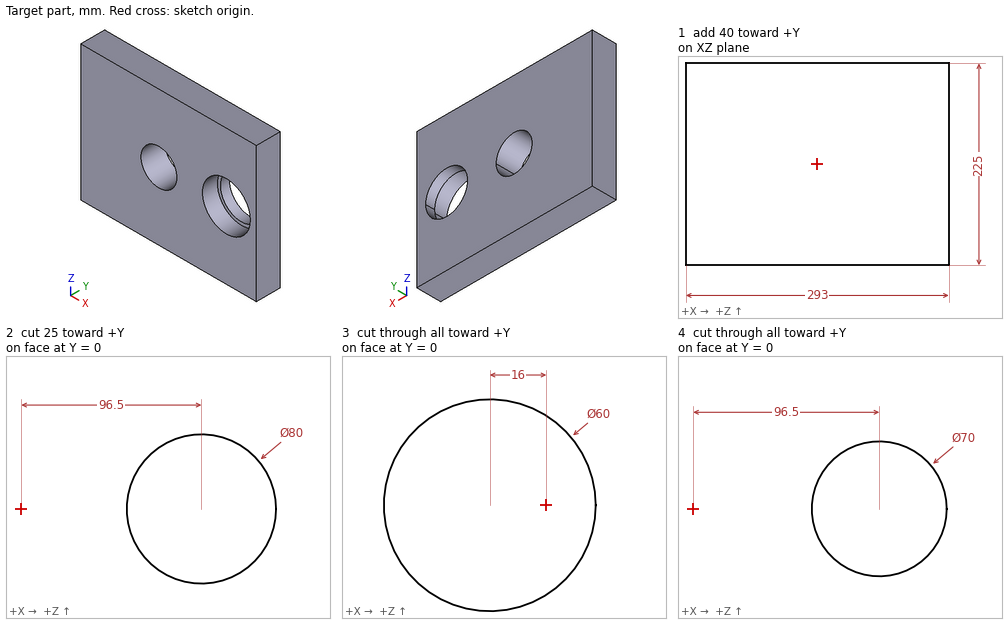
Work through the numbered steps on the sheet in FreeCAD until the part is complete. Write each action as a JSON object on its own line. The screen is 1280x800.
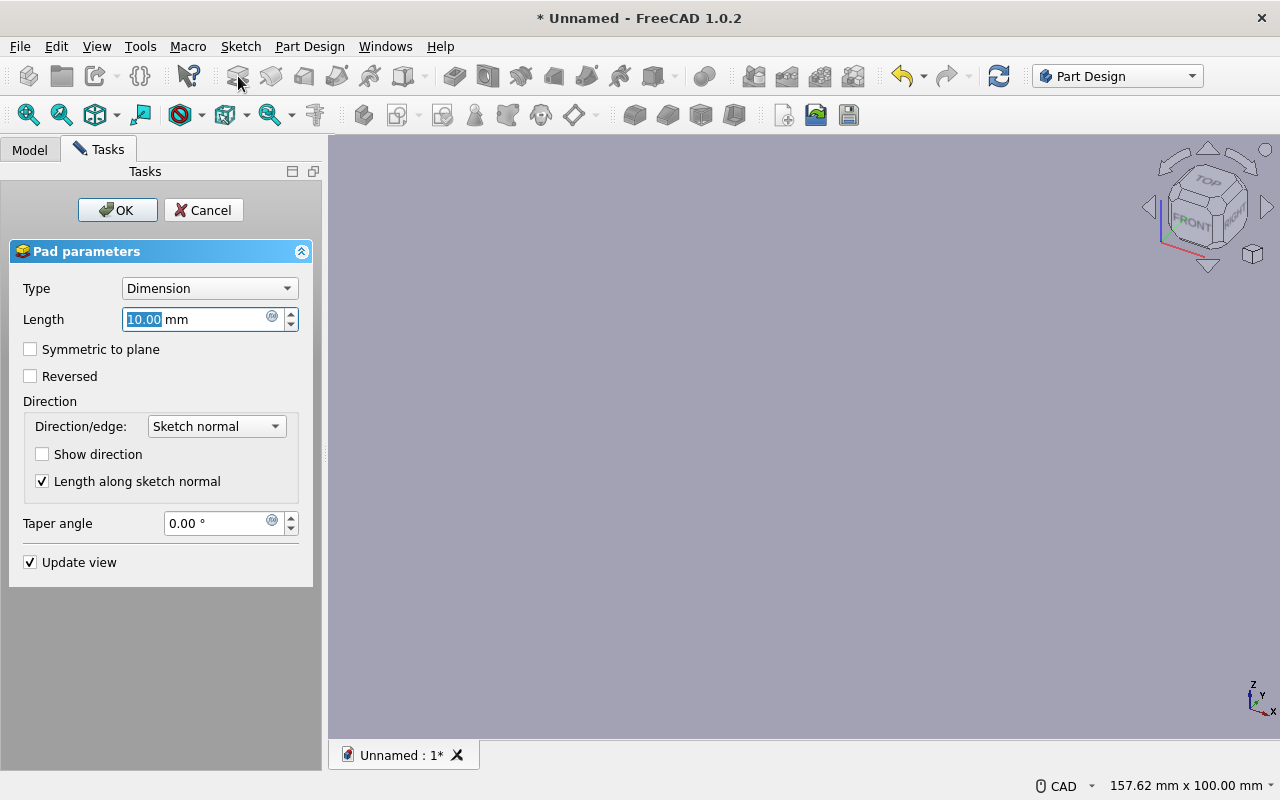
{"action": "type", "text": "40"}
{"action": "key", "text": "Tab"}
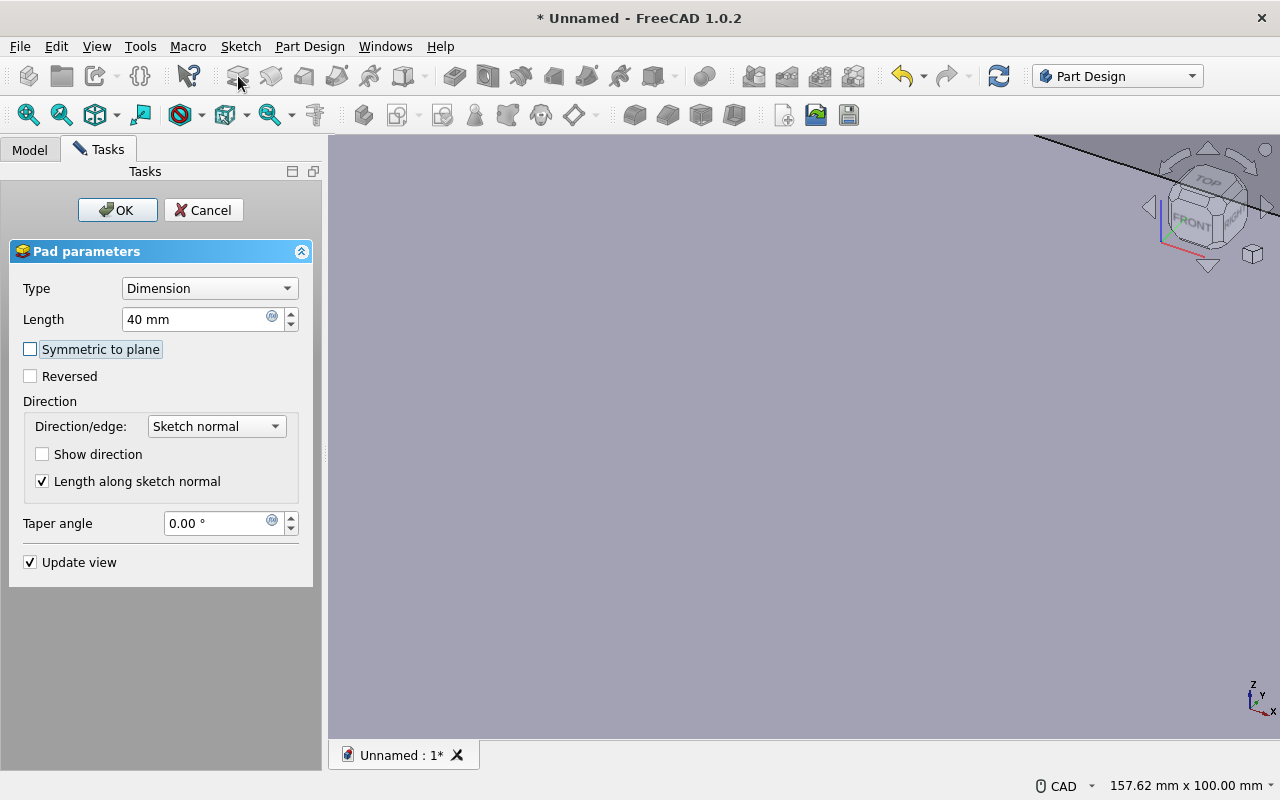
{"action": "left_click", "coordinate": [31, 376]}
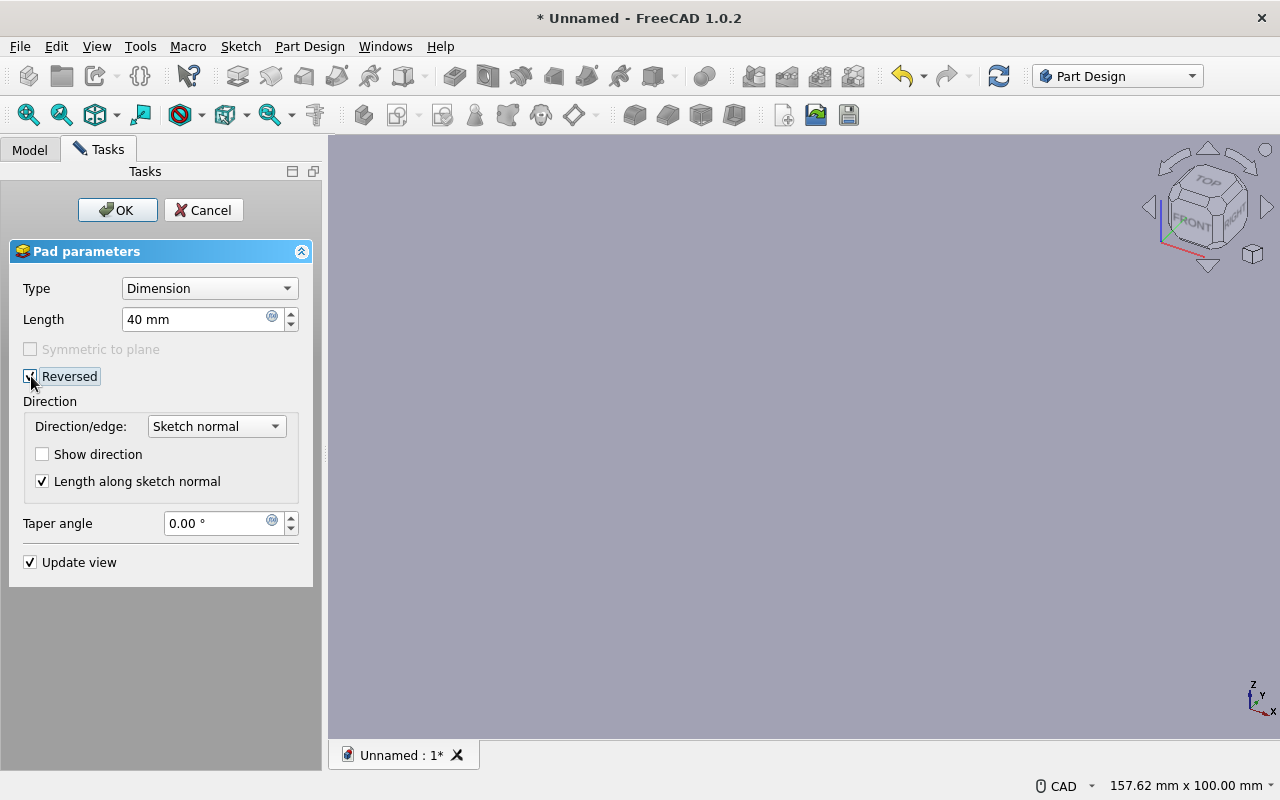
{"action": "left_click", "coordinate": [118, 210]}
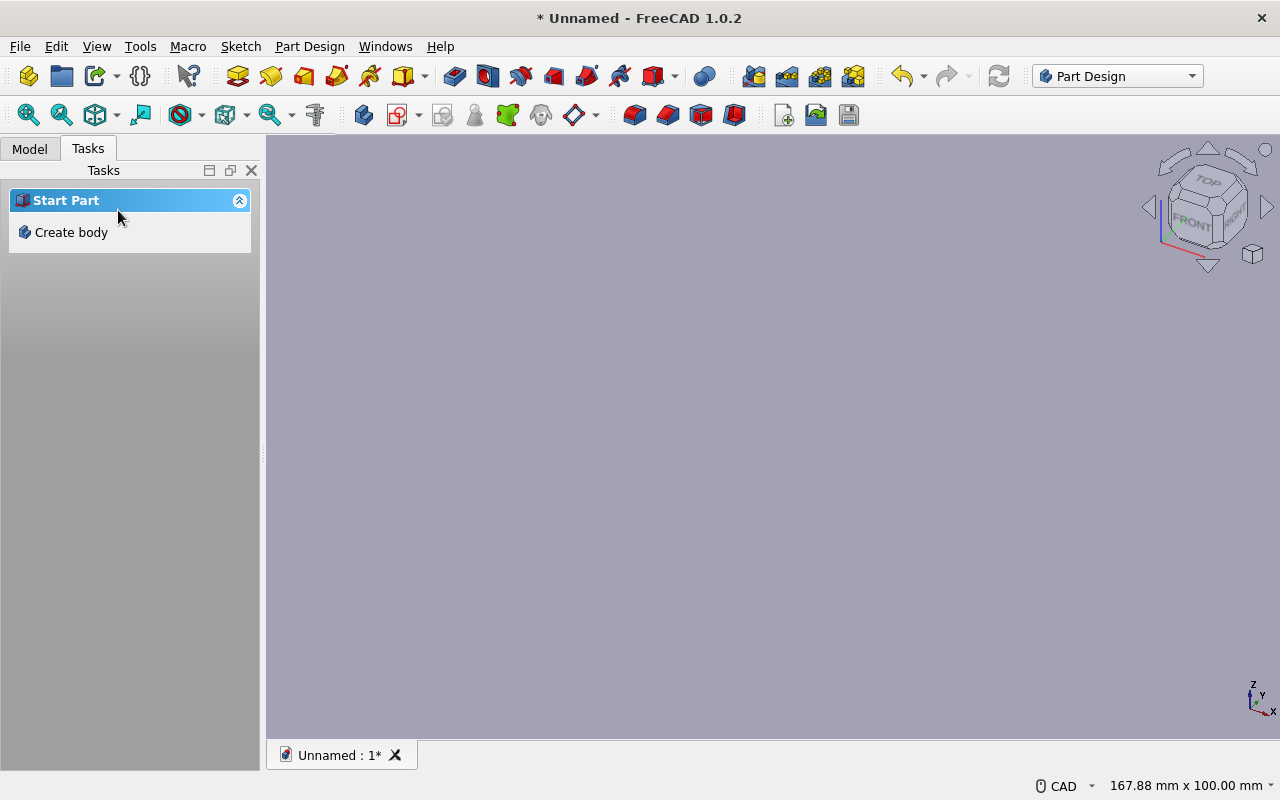
{"action": "left_click", "coordinate": [29, 116]}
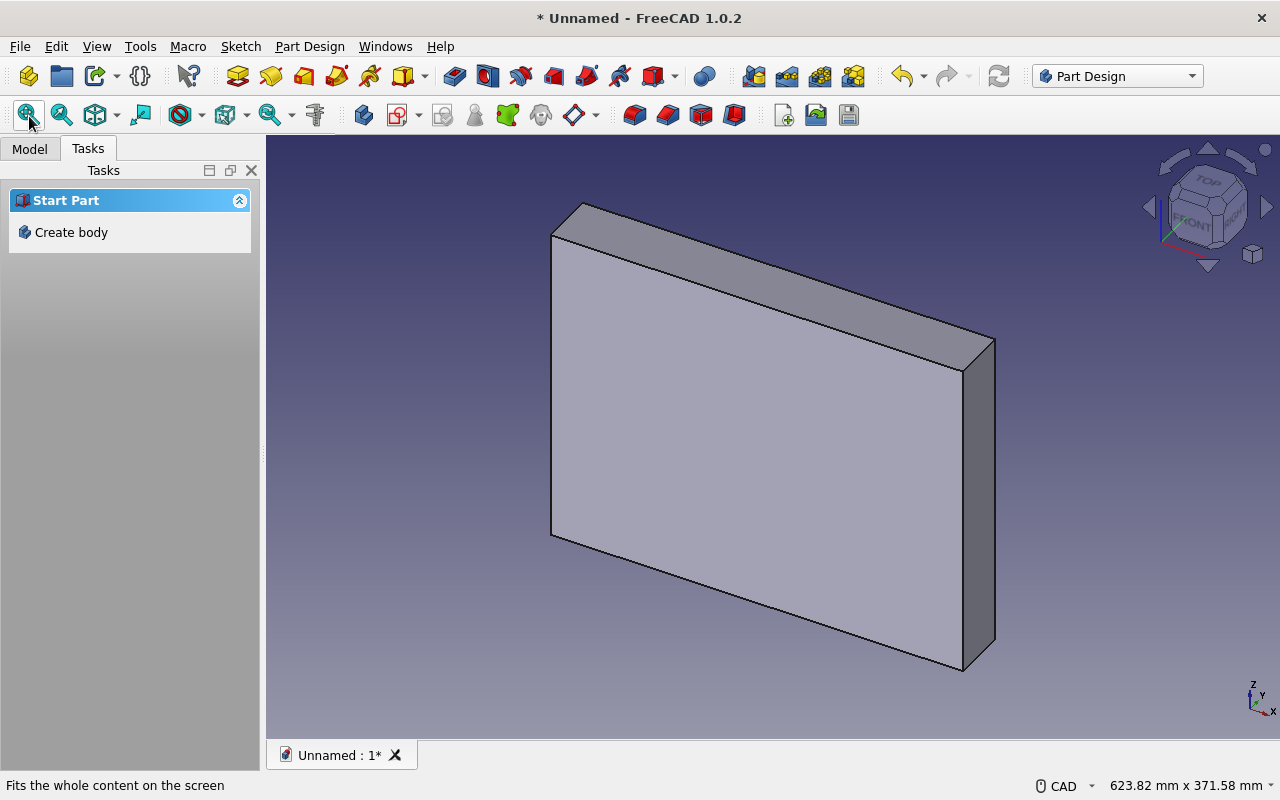
{"action": "left_click", "coordinate": [757, 452]}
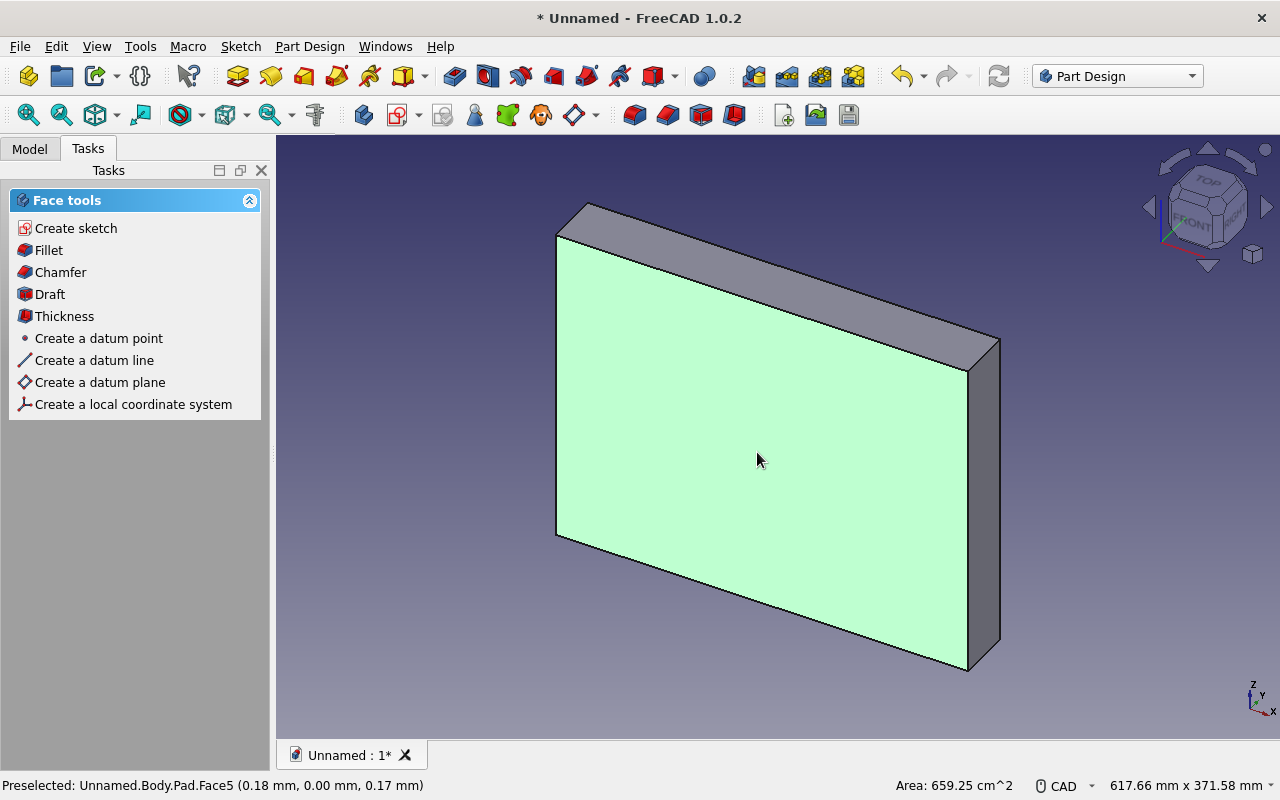
{"action": "left_click", "coordinate": [396, 116]}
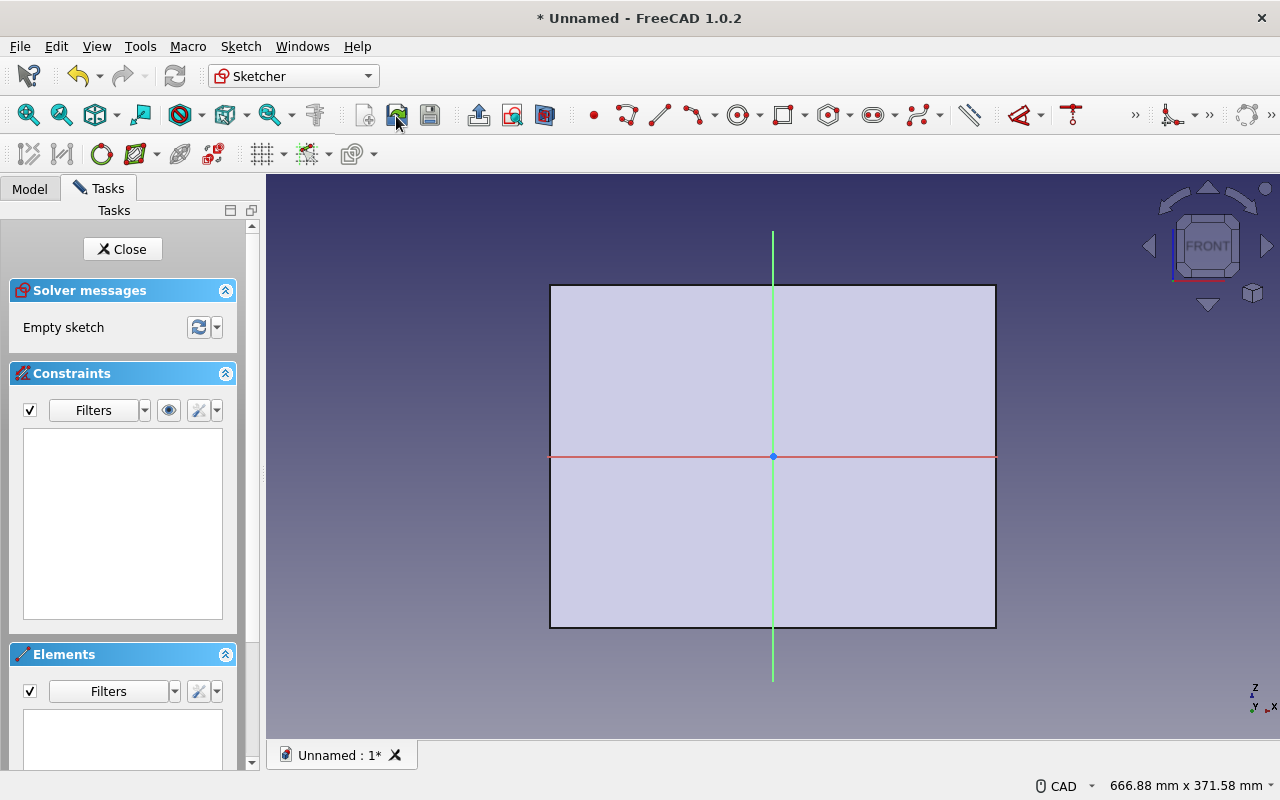
{"action": "scroll", "coordinate": [977, 457], "scroll_direction": "up", "scroll_amount": 5}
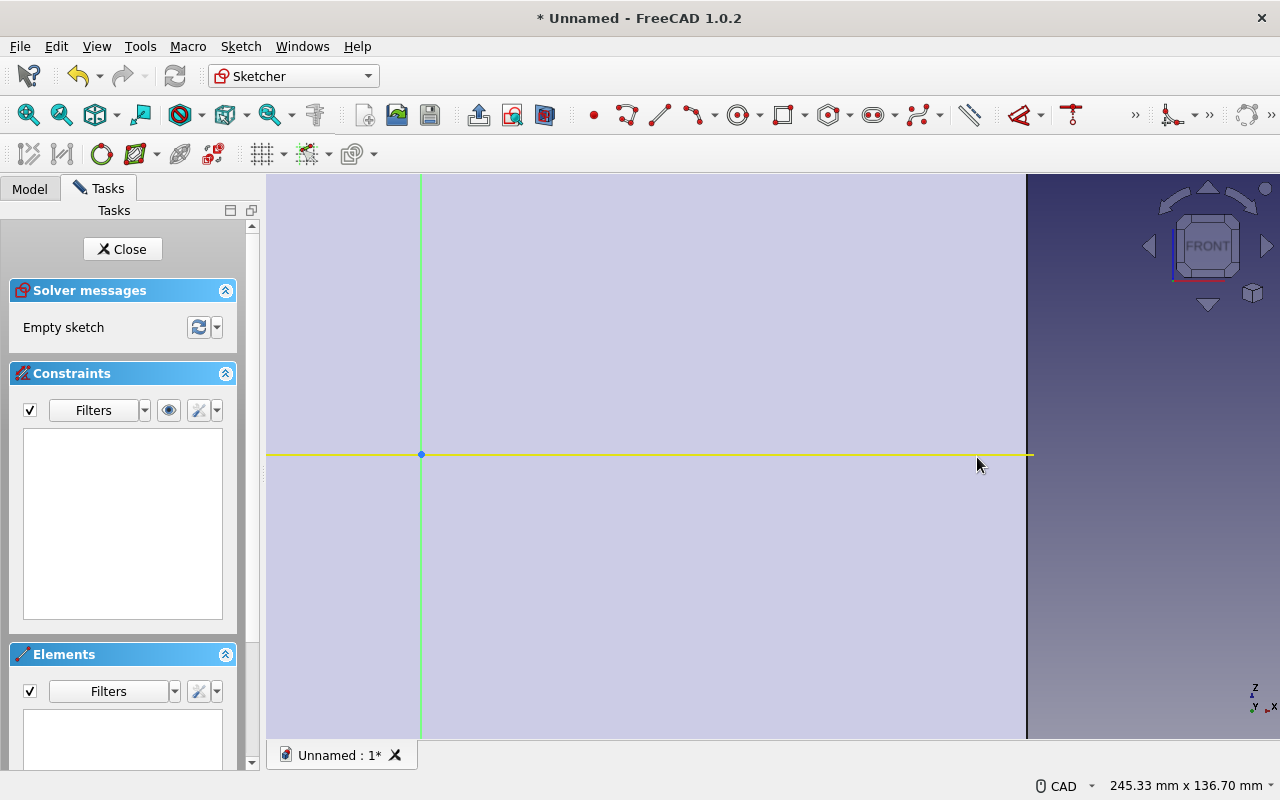
{"action": "left_click", "coordinate": [738, 116]}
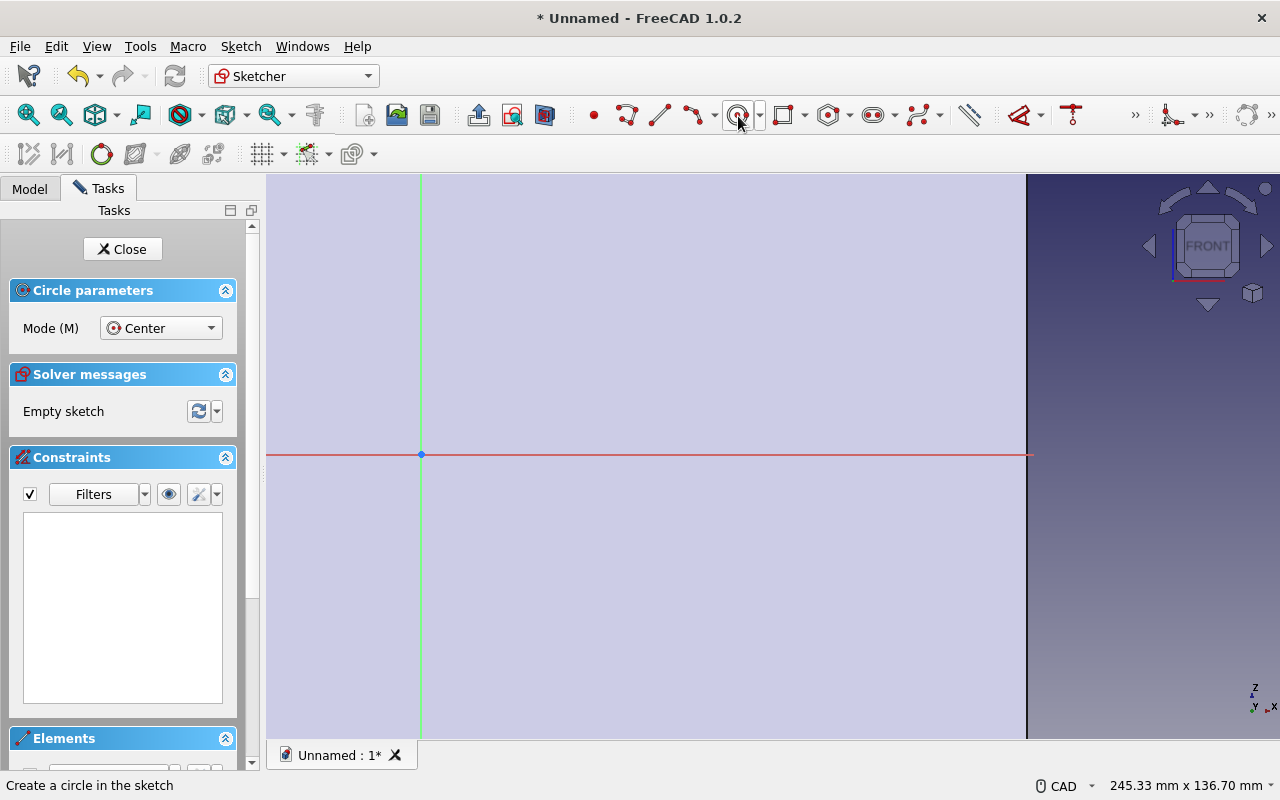
{"action": "left_click", "coordinate": [820, 455]}
{"action": "mouse_move", "coordinate": [937, 338]}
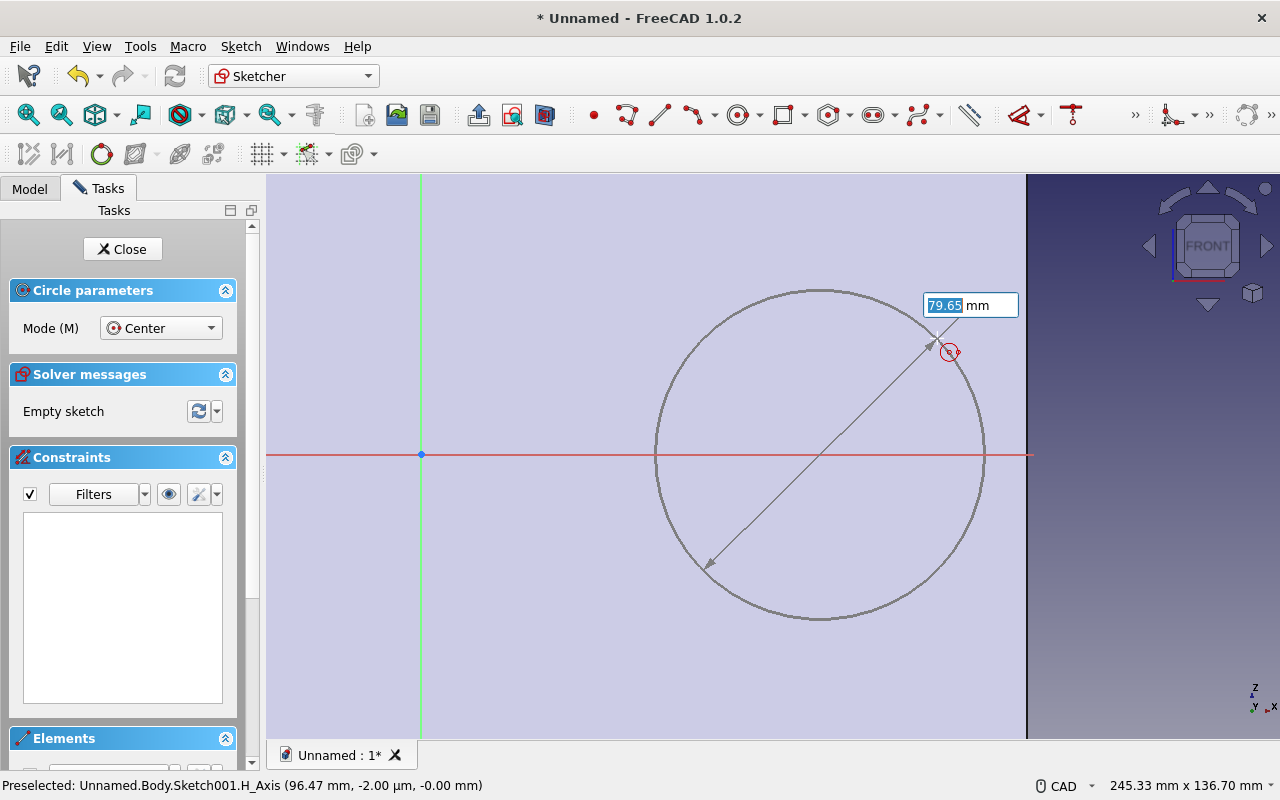
{"action": "type", "text": "80"}
{"action": "key", "text": "Return"}
{"action": "key", "text": "Escape"}